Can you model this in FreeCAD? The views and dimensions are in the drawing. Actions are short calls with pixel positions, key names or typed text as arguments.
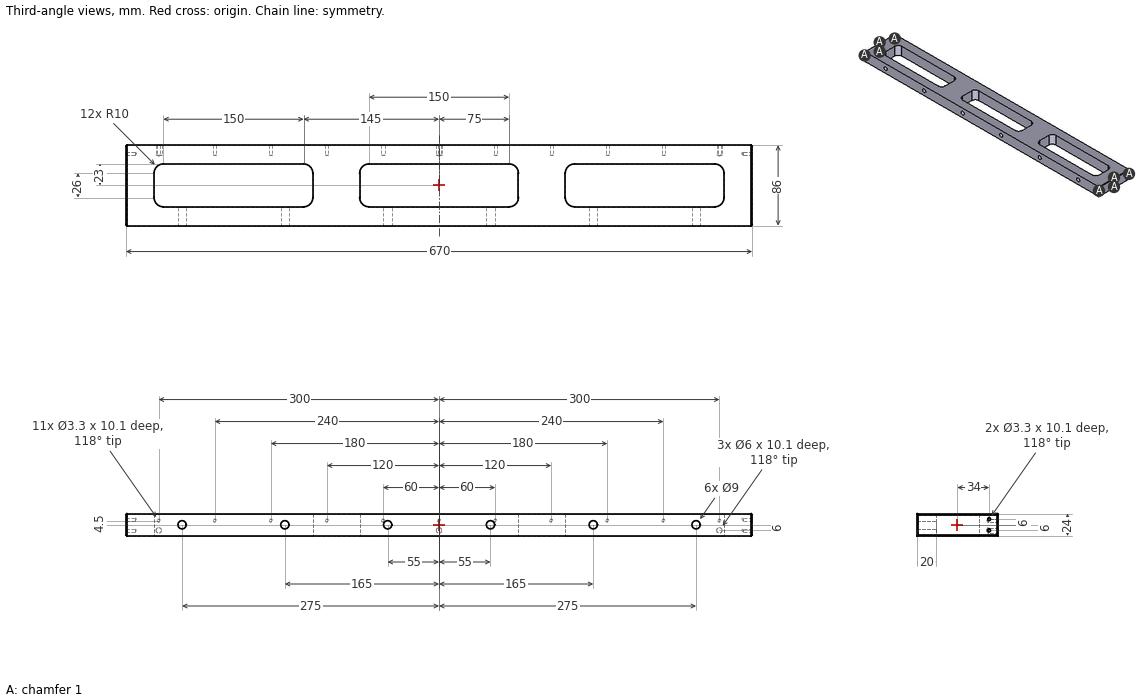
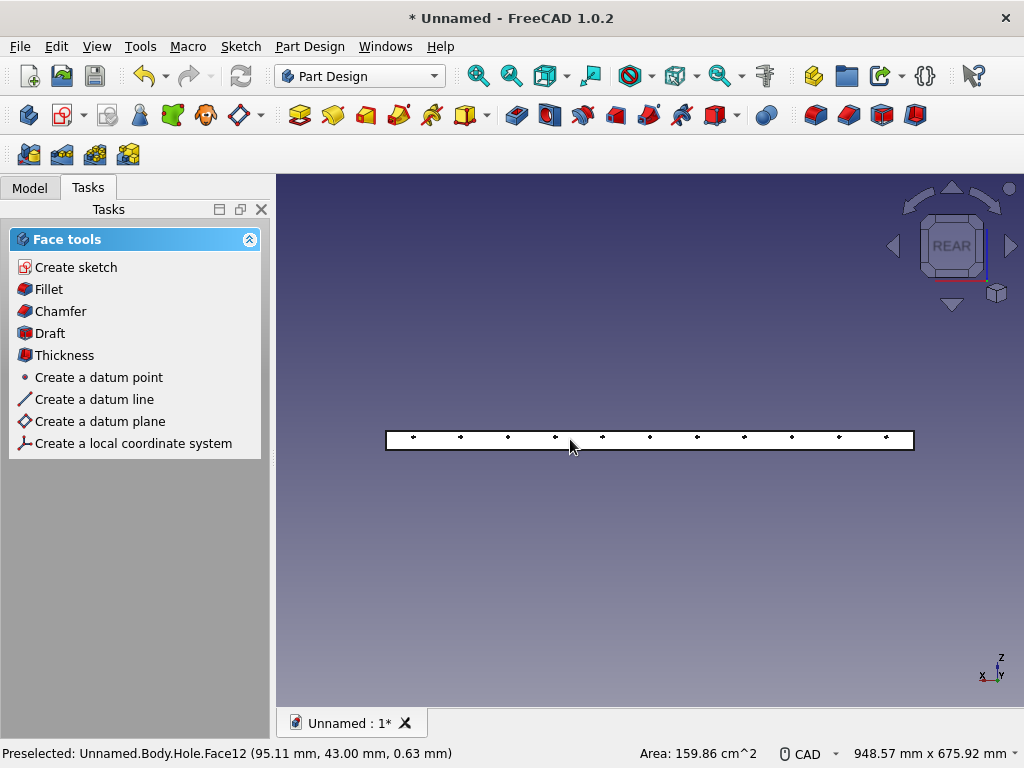
click(62, 116)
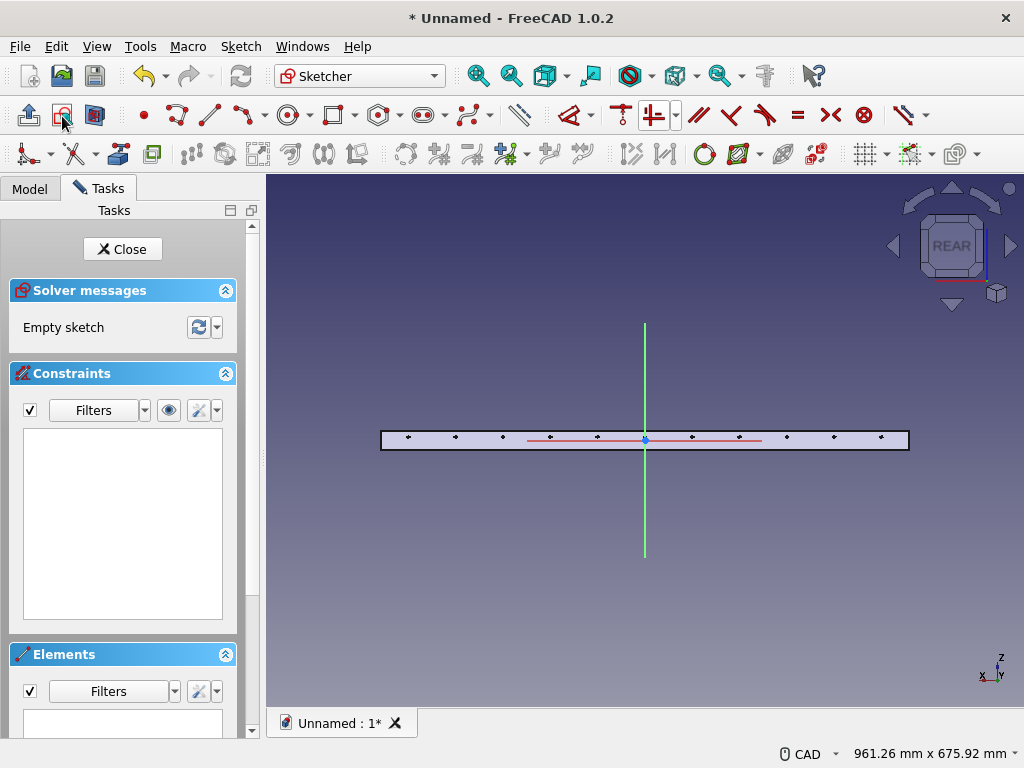
scroll(294, 424, down, 1)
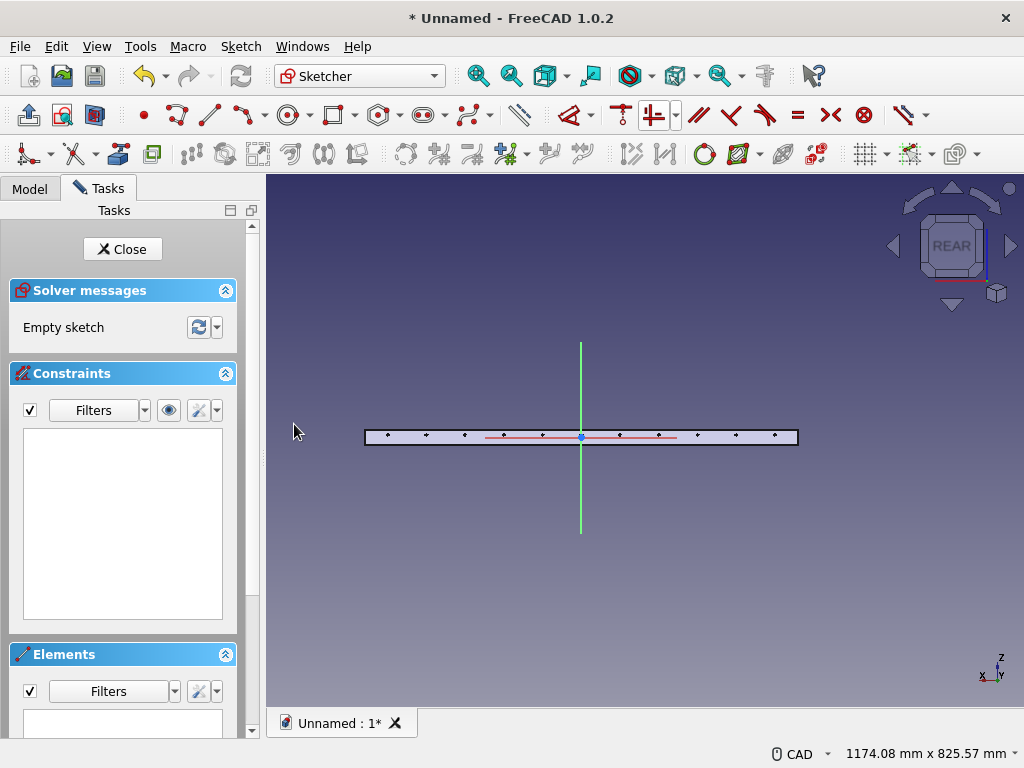
key(g)
key(c)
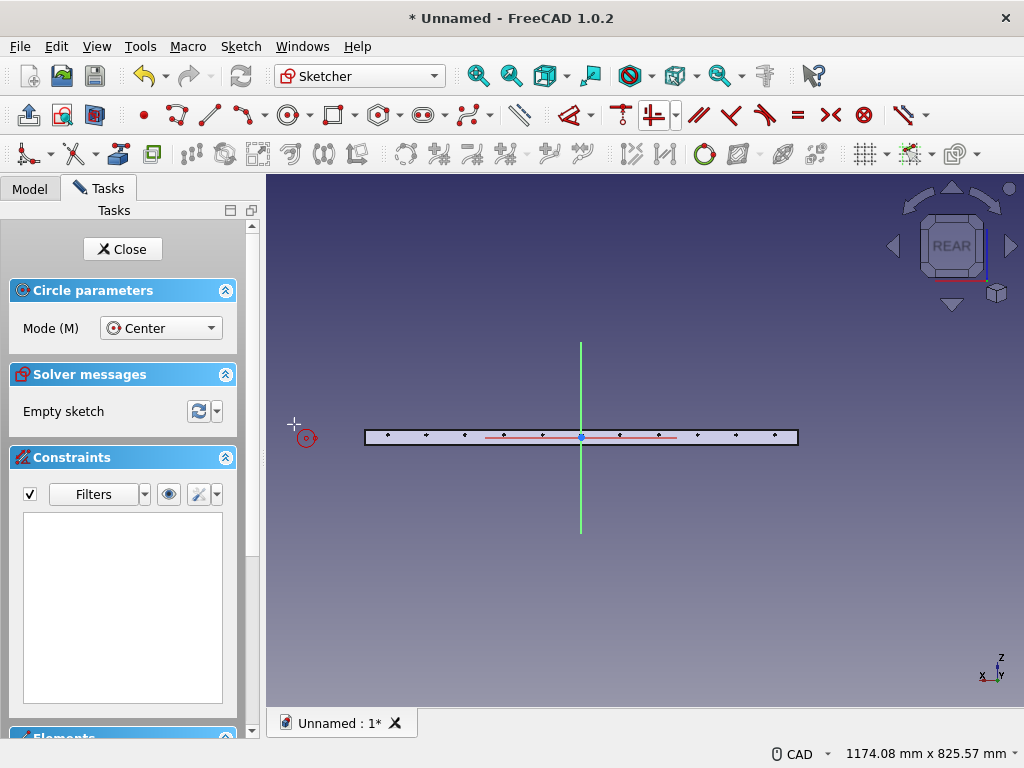
scroll(388, 441, up, 13)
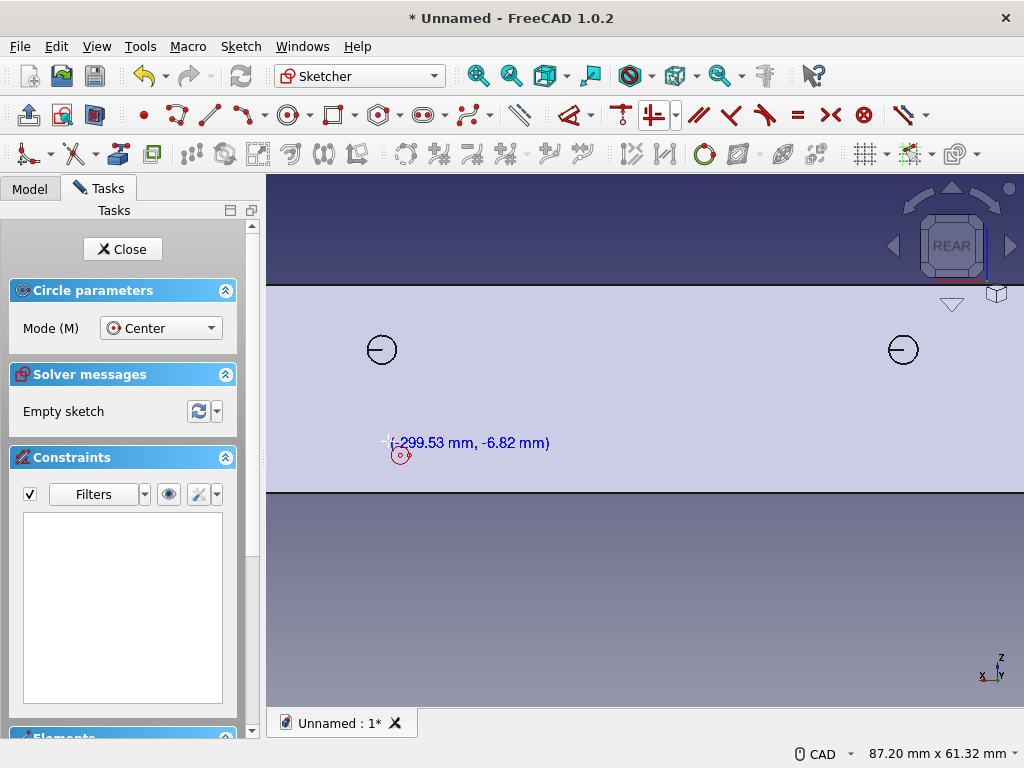
scroll(383, 442, down, 13)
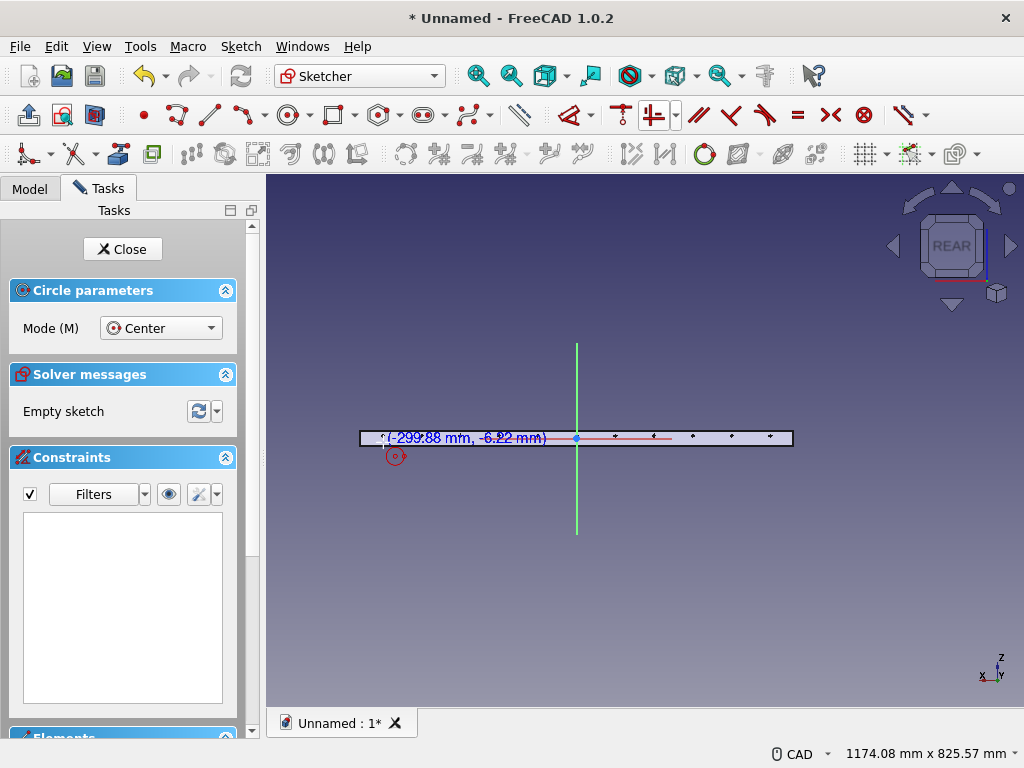
scroll(383, 442, up, 8)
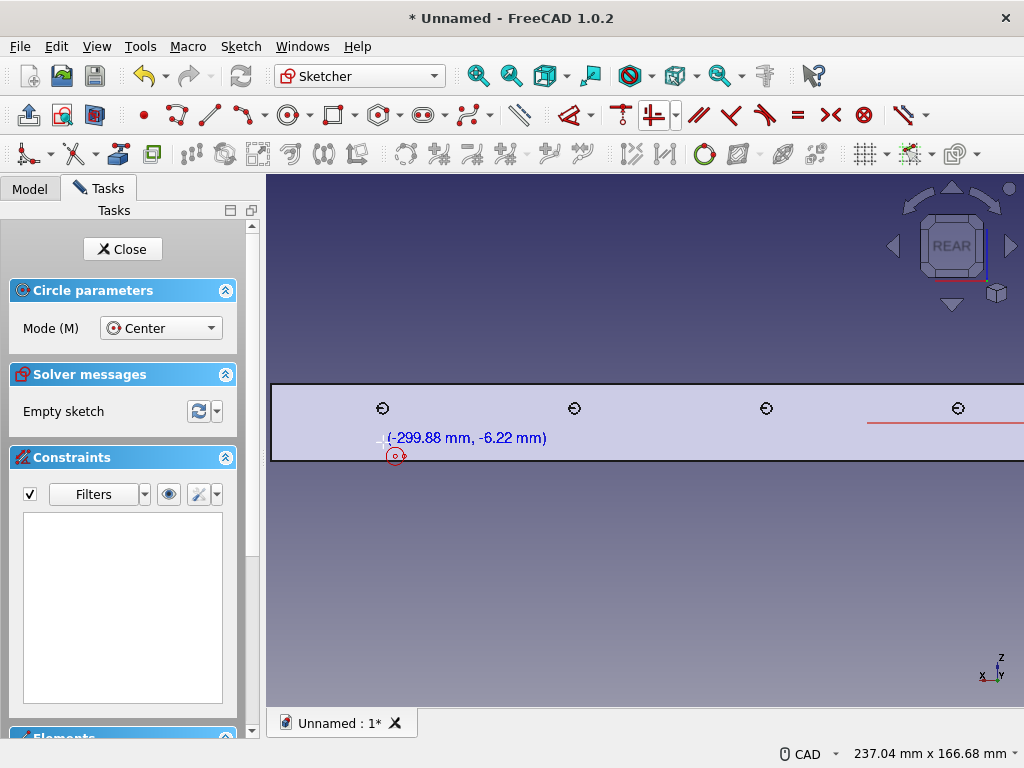
click(383, 442)
move(389, 449)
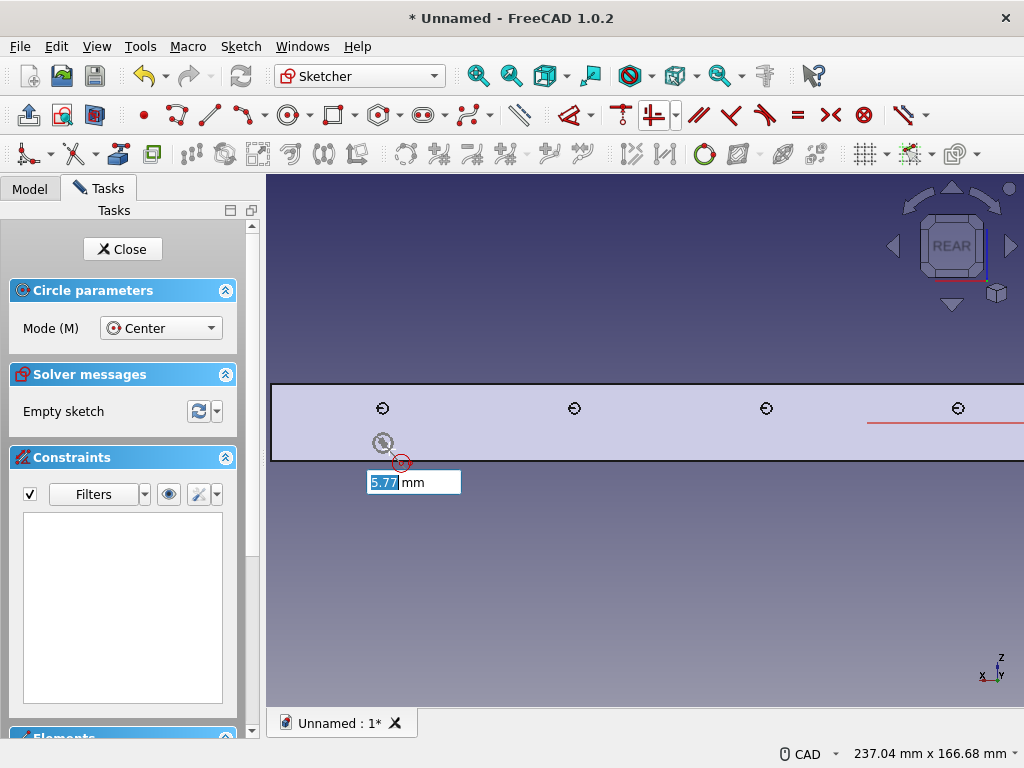
text(6)
key(Return)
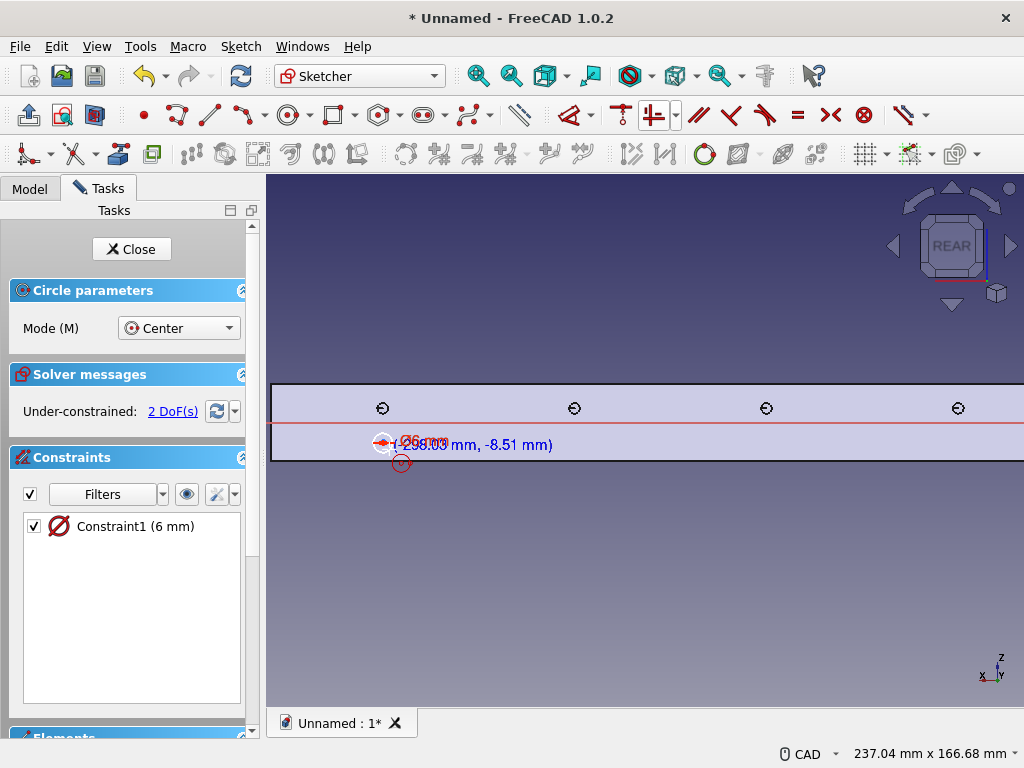
scroll(383, 441, down, 8)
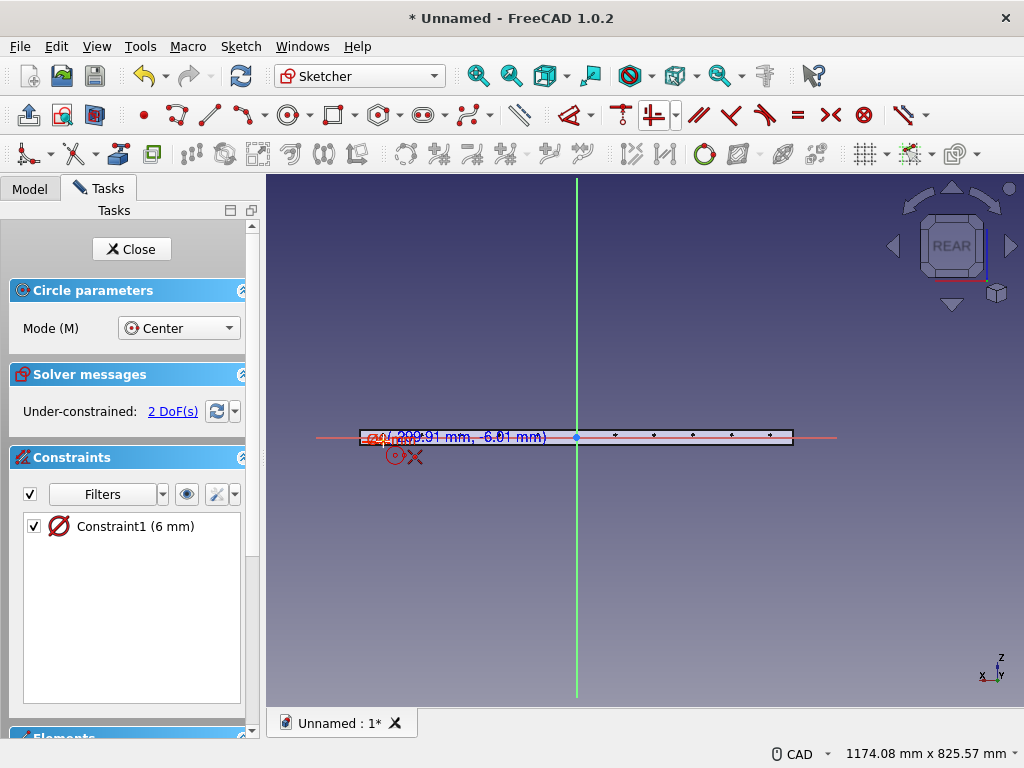
scroll(770, 442, up, 13)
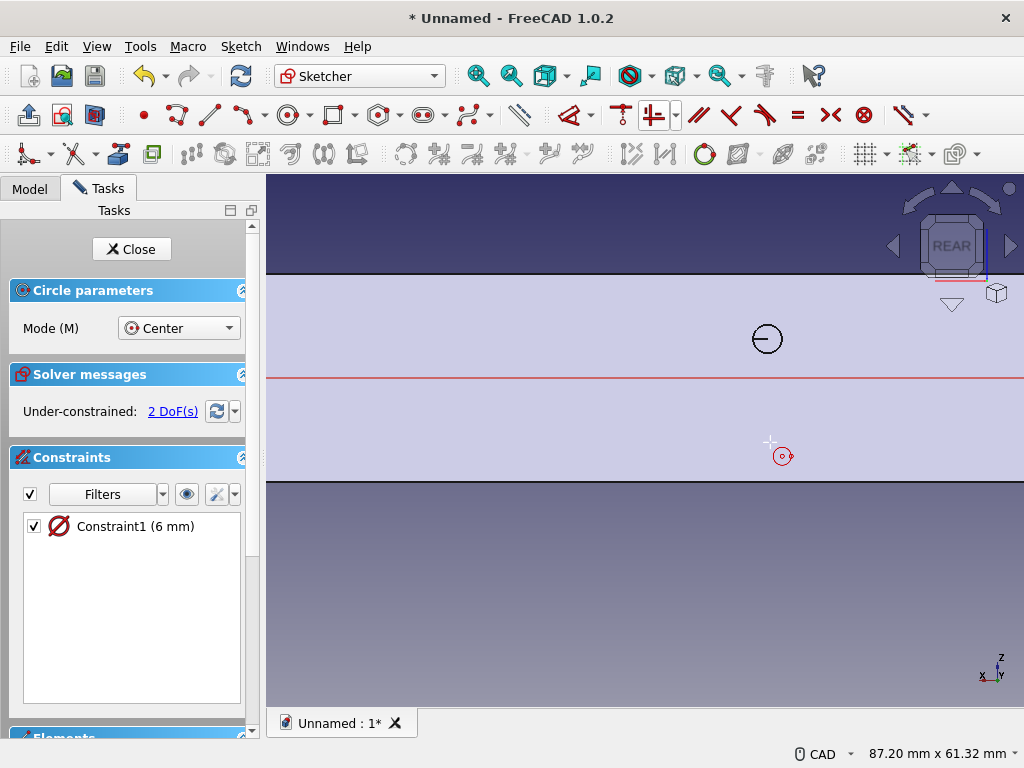
scroll(770, 442, down, 13)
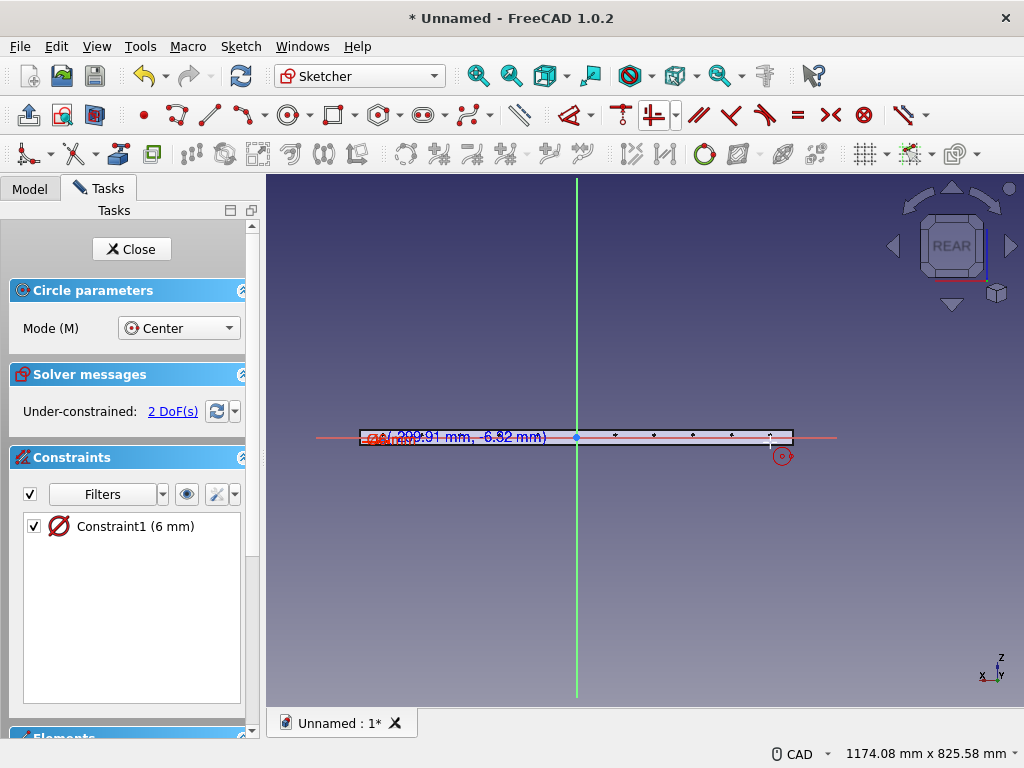
scroll(770, 442, up, 8)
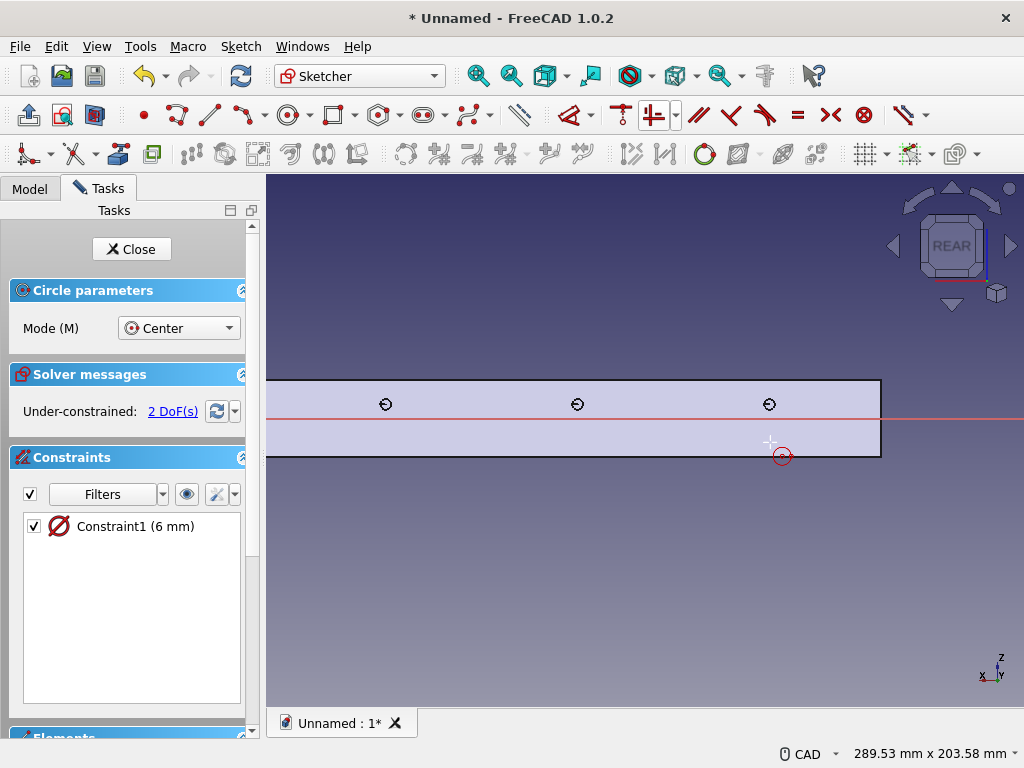
click(769, 438)
move(776, 445)